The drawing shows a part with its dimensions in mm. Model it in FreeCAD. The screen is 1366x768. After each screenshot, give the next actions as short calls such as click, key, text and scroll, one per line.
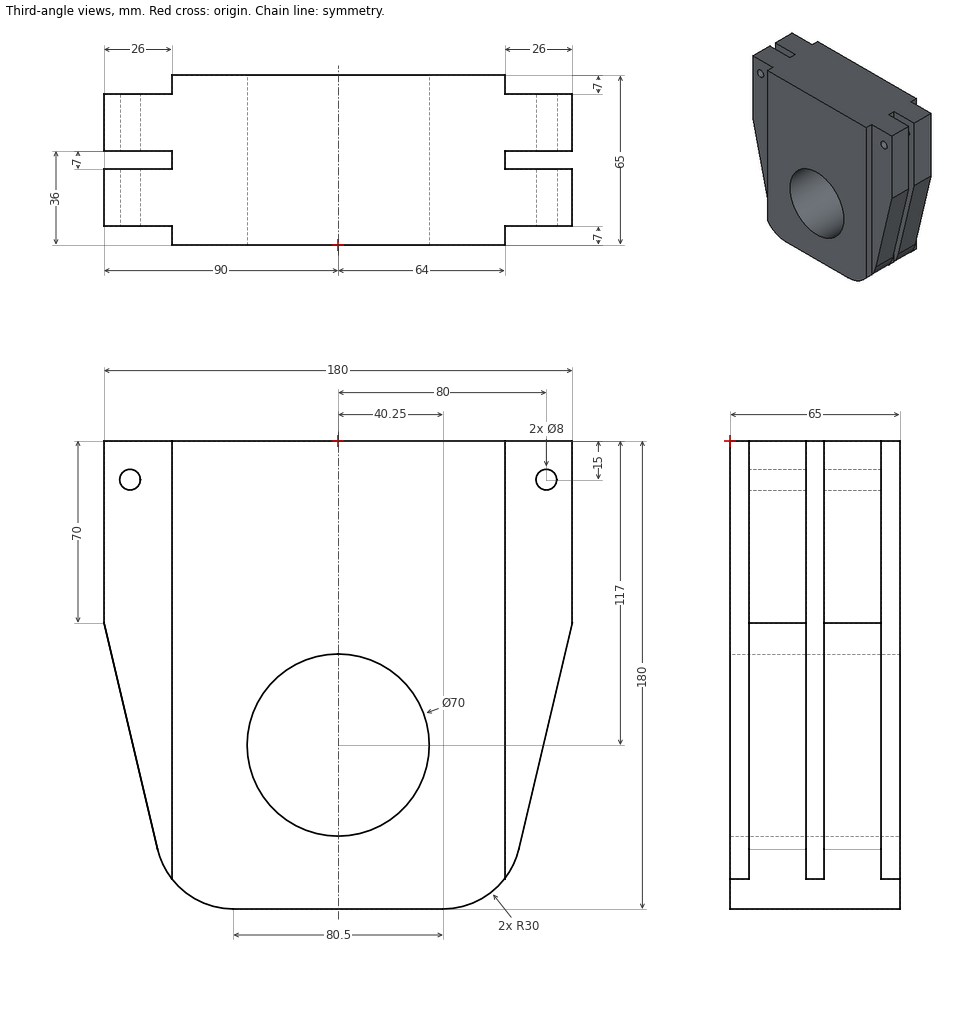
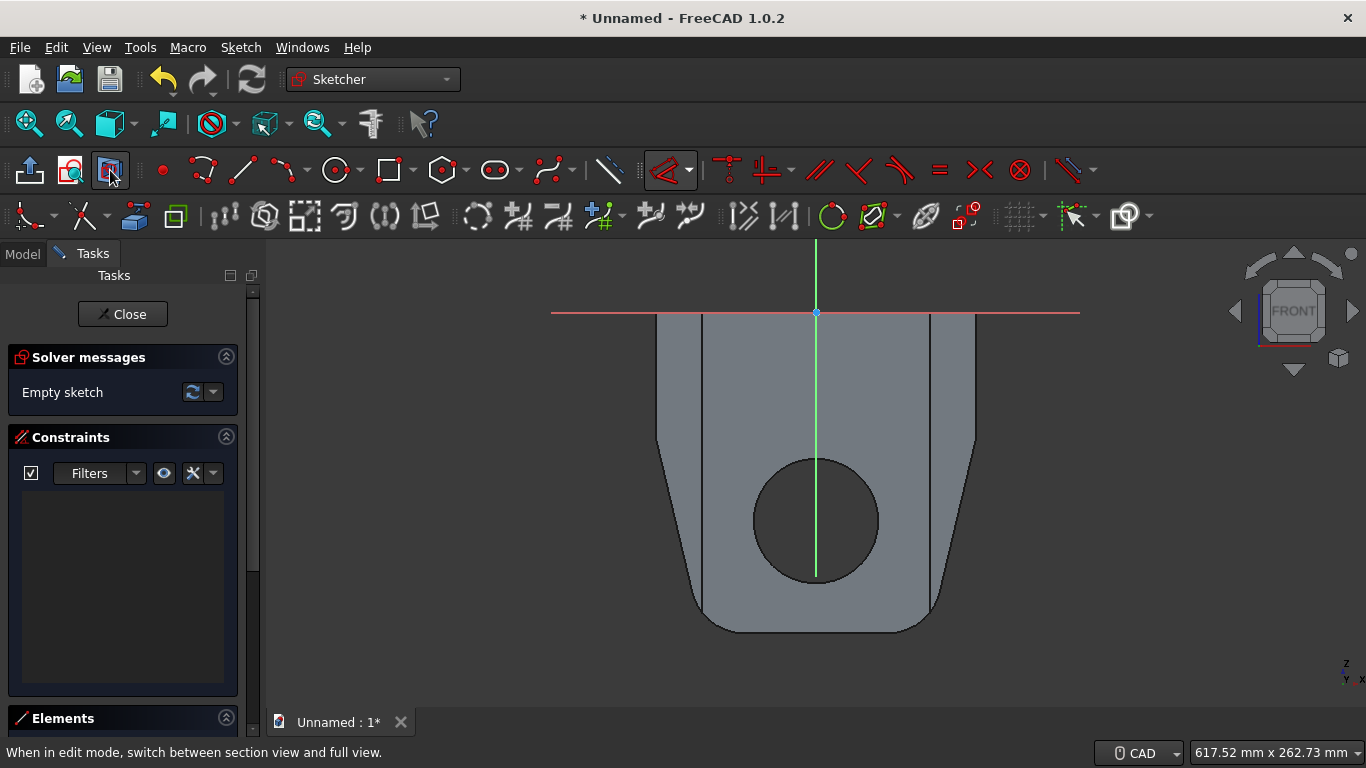
scroll(872, 267, up, 4)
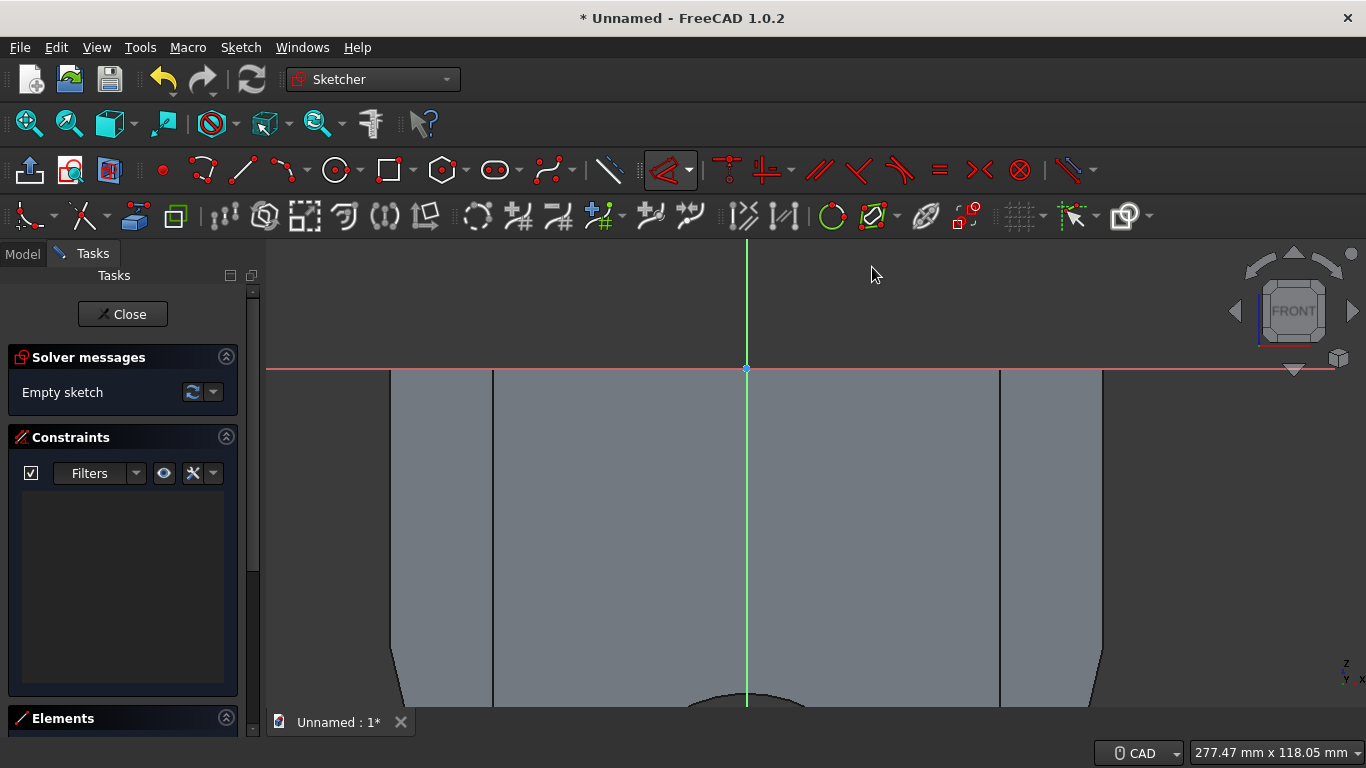
click(336, 170)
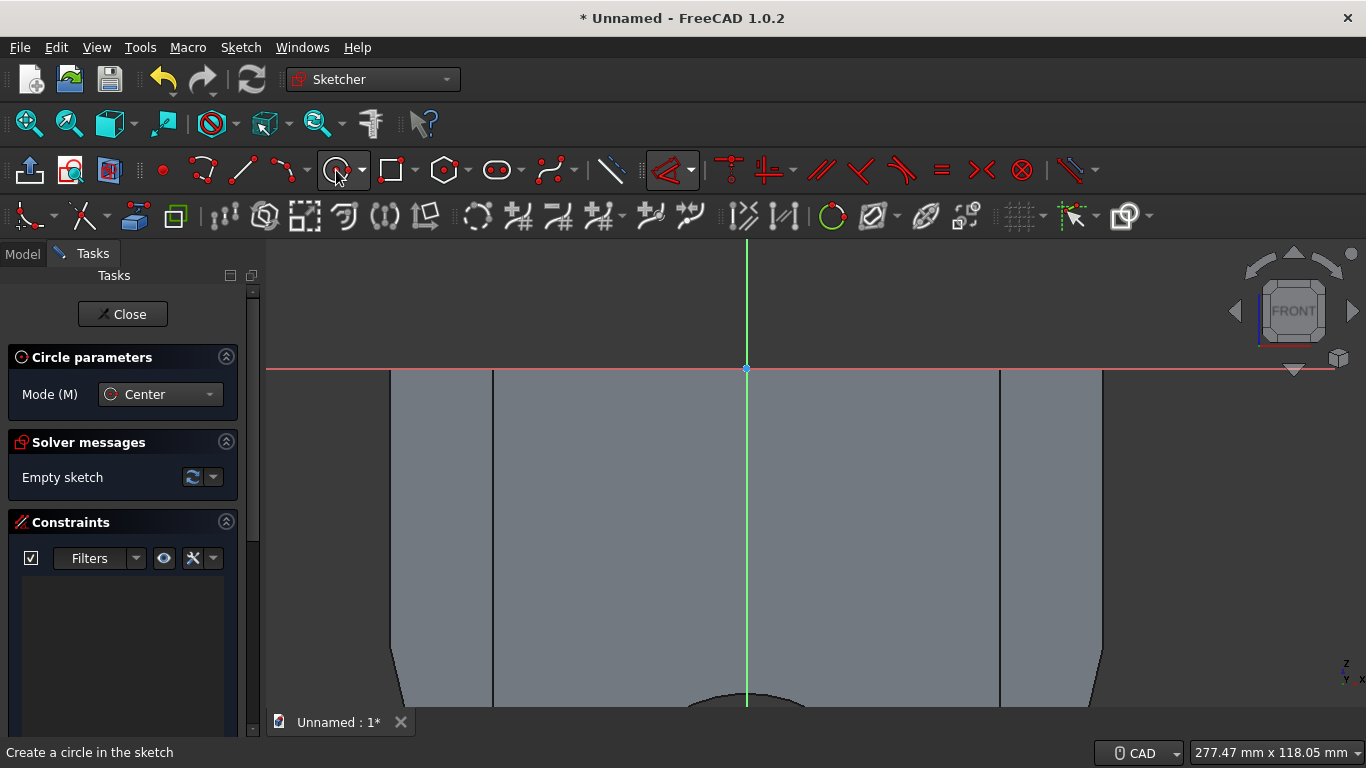
scroll(1064, 428, up, 2)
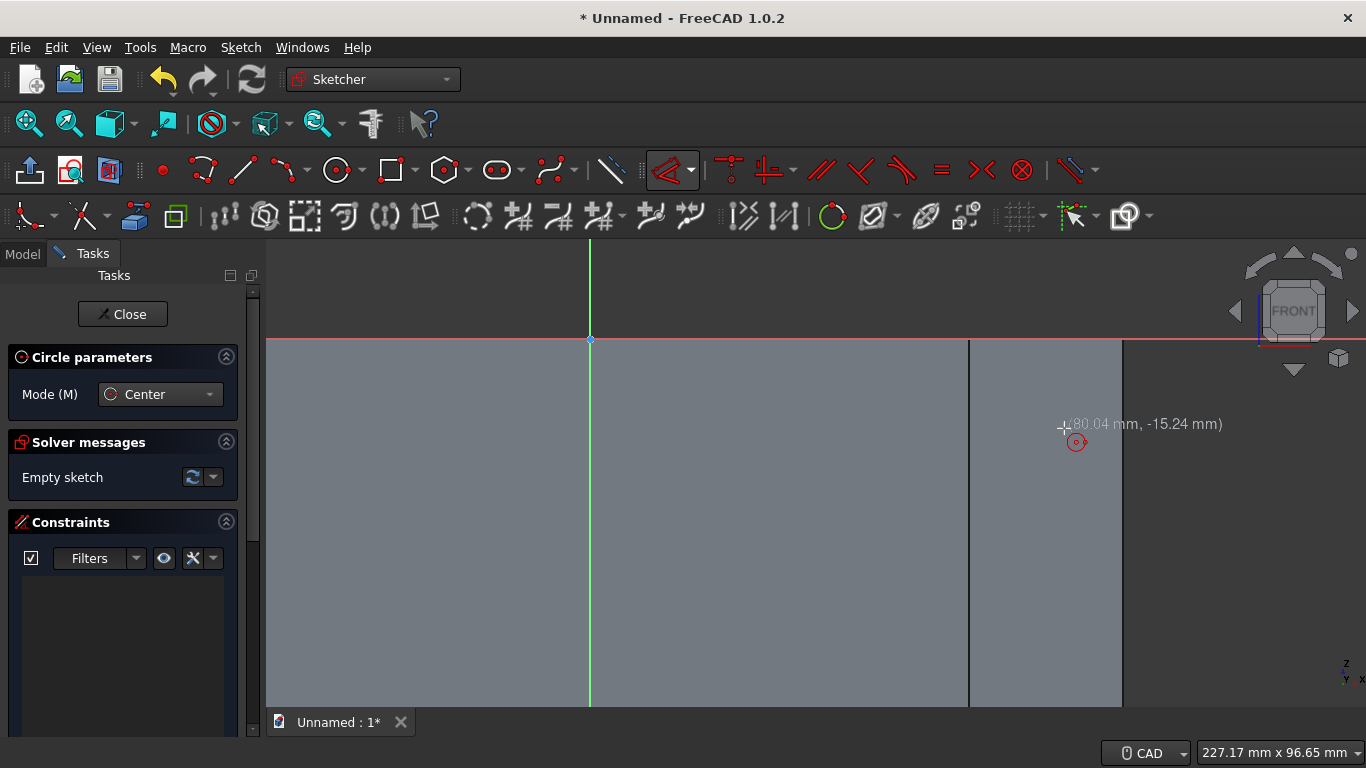
click(1063, 428)
move(1080, 411)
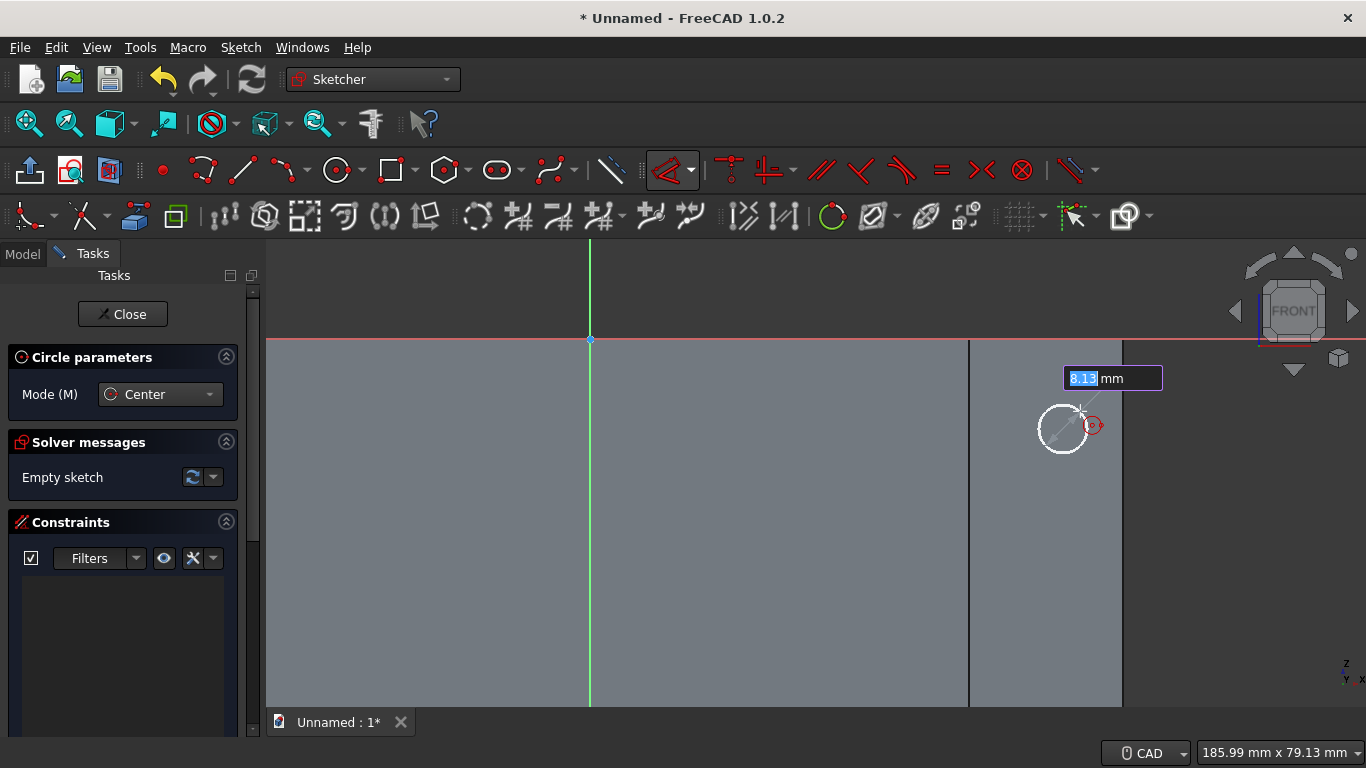
text(8)
key(Return)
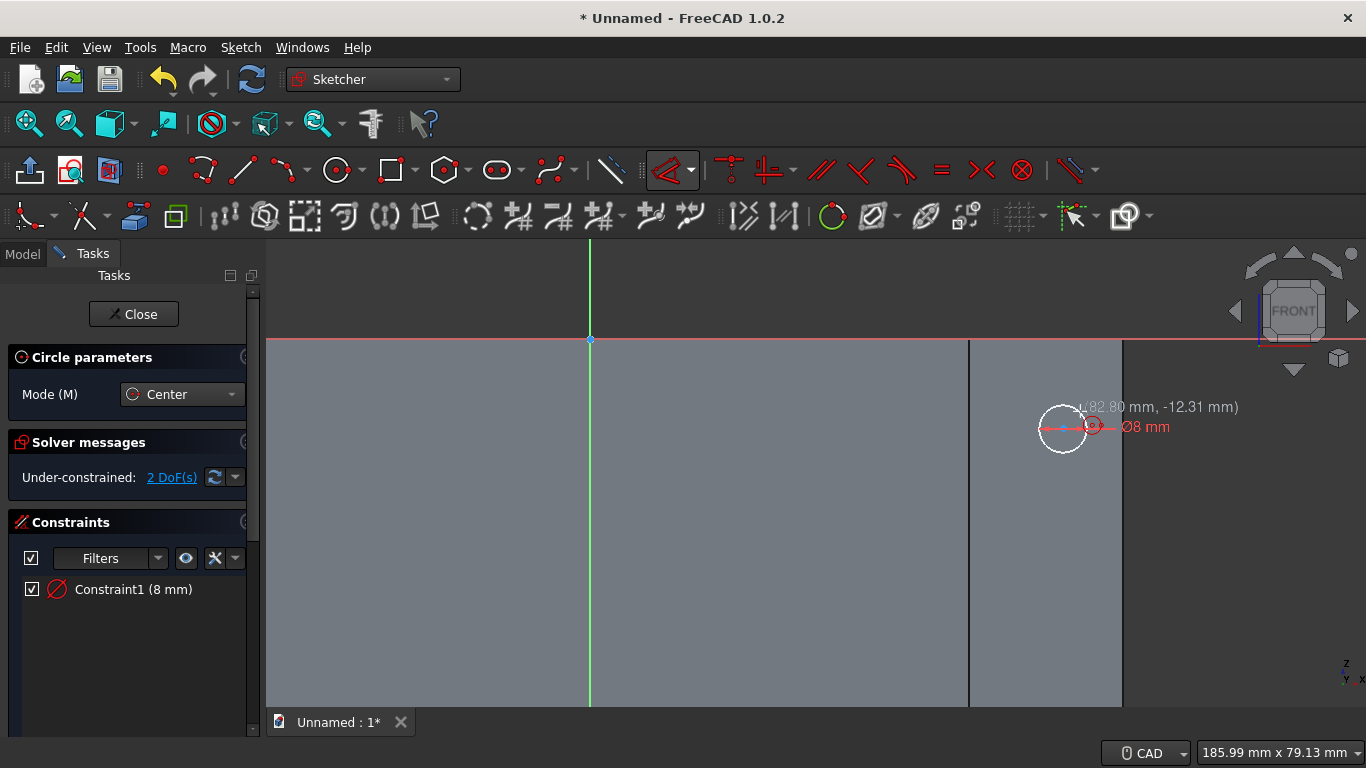
scroll(1067, 631, down, 2)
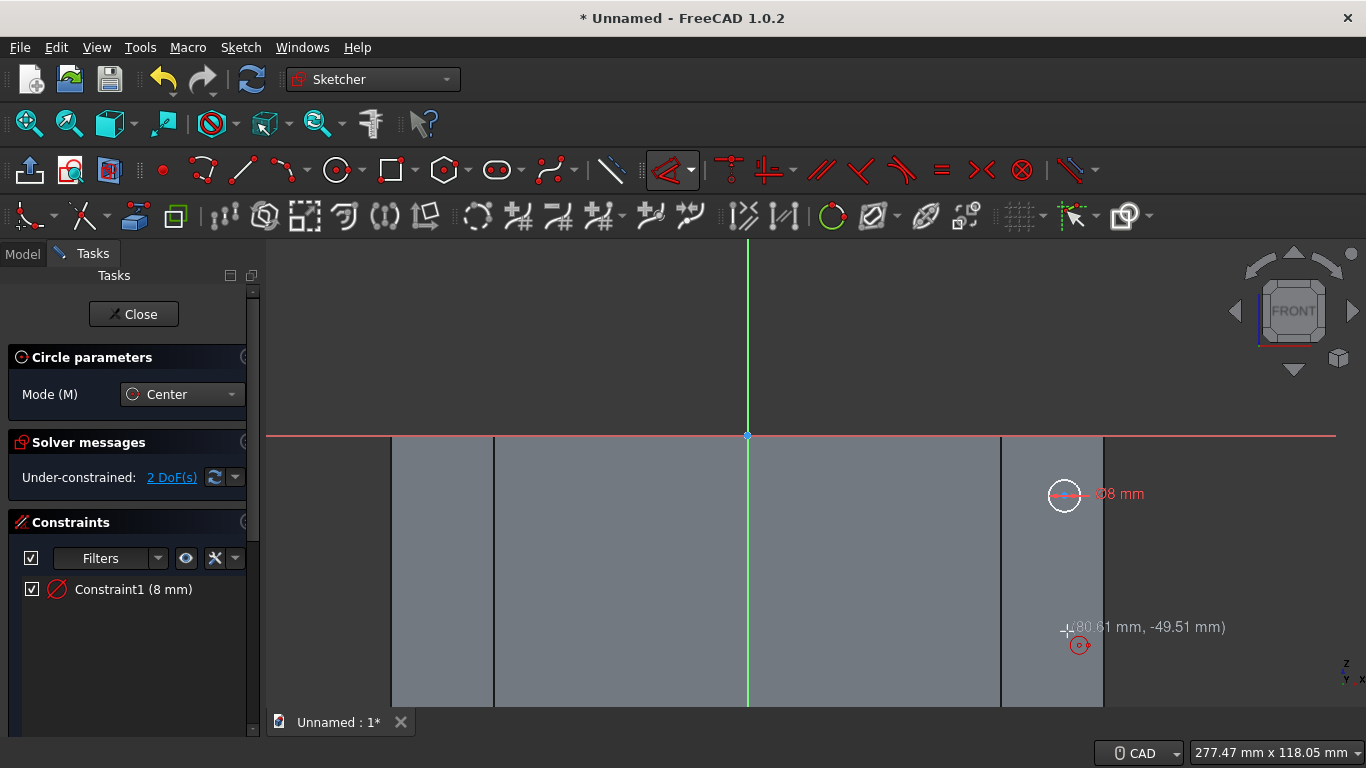
scroll(431, 495, up, 2)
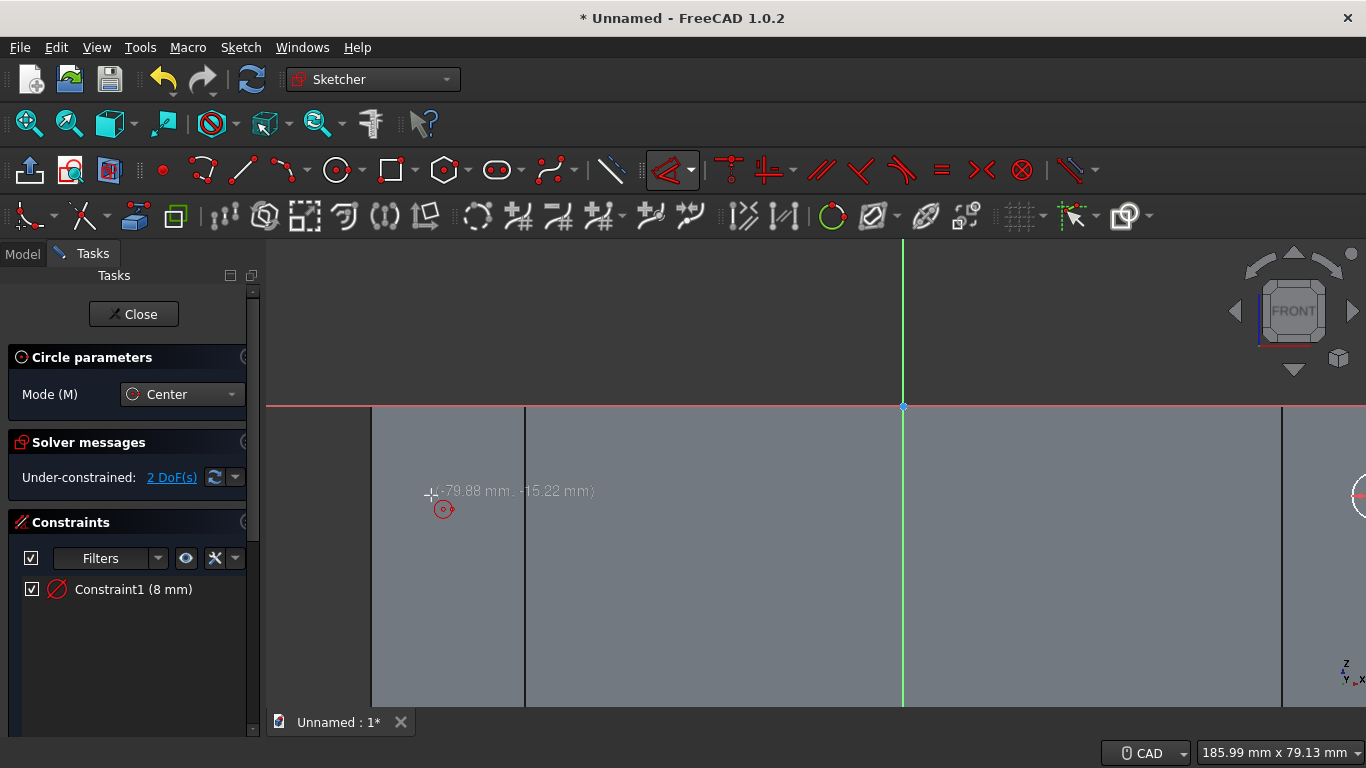
click(430, 495)
move(447, 478)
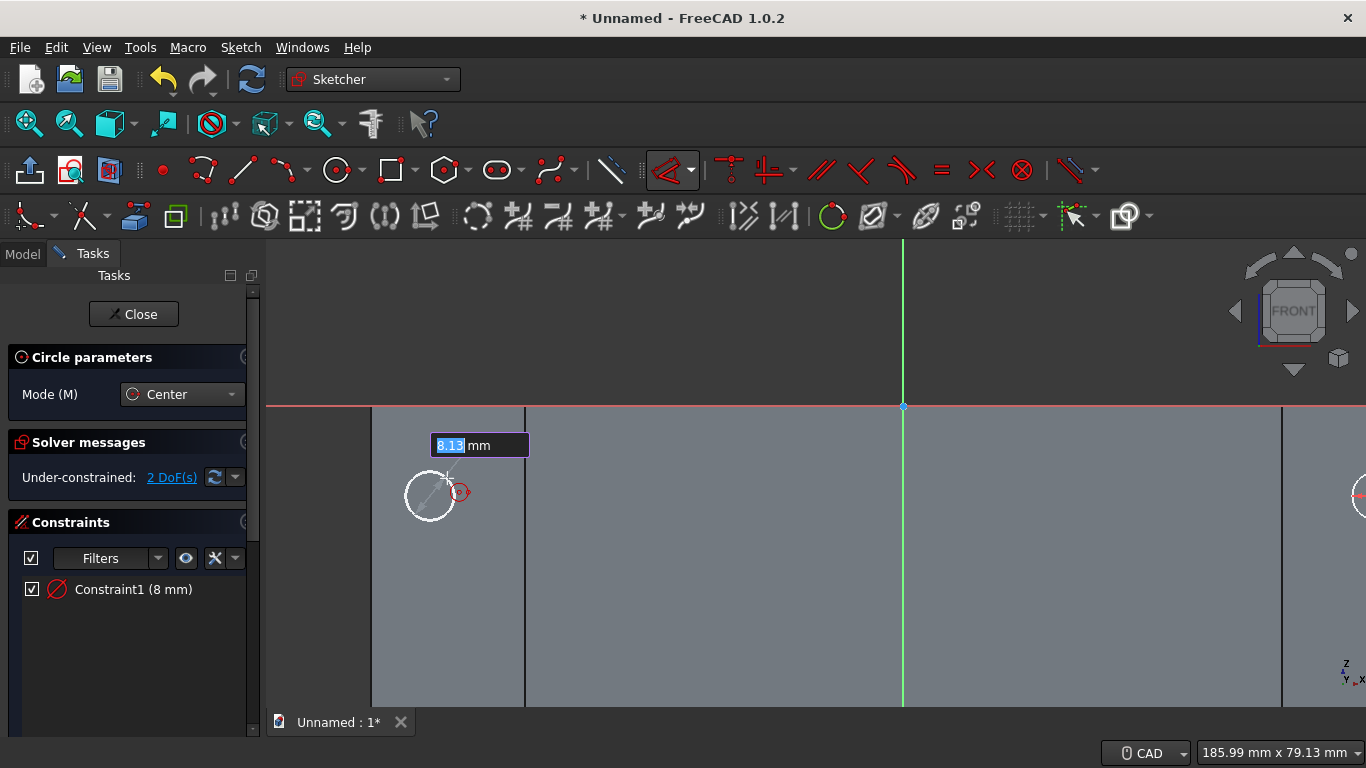
text(8)
key(Return)
key(Escape)